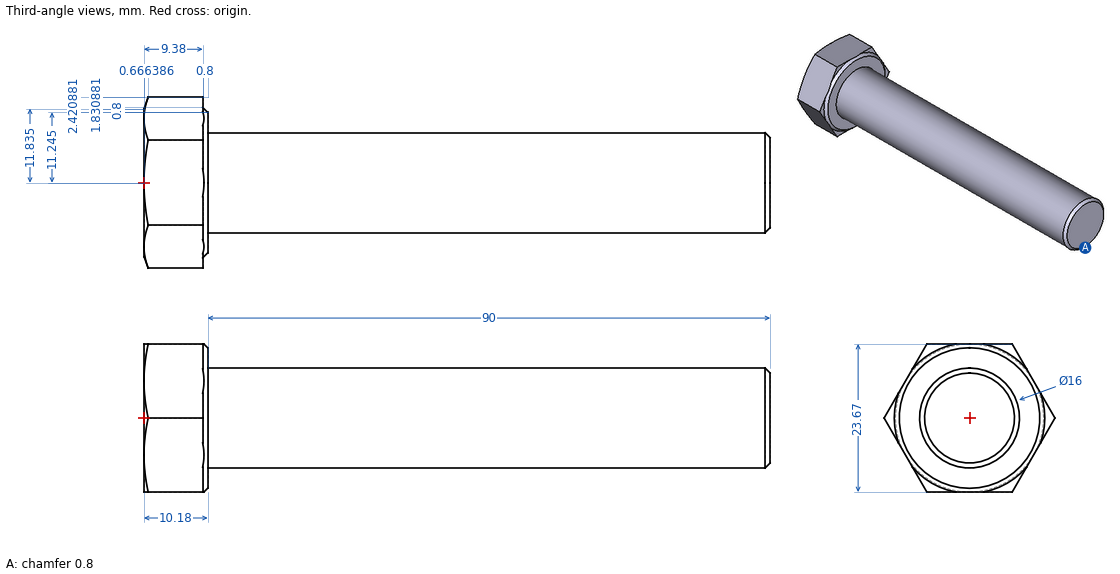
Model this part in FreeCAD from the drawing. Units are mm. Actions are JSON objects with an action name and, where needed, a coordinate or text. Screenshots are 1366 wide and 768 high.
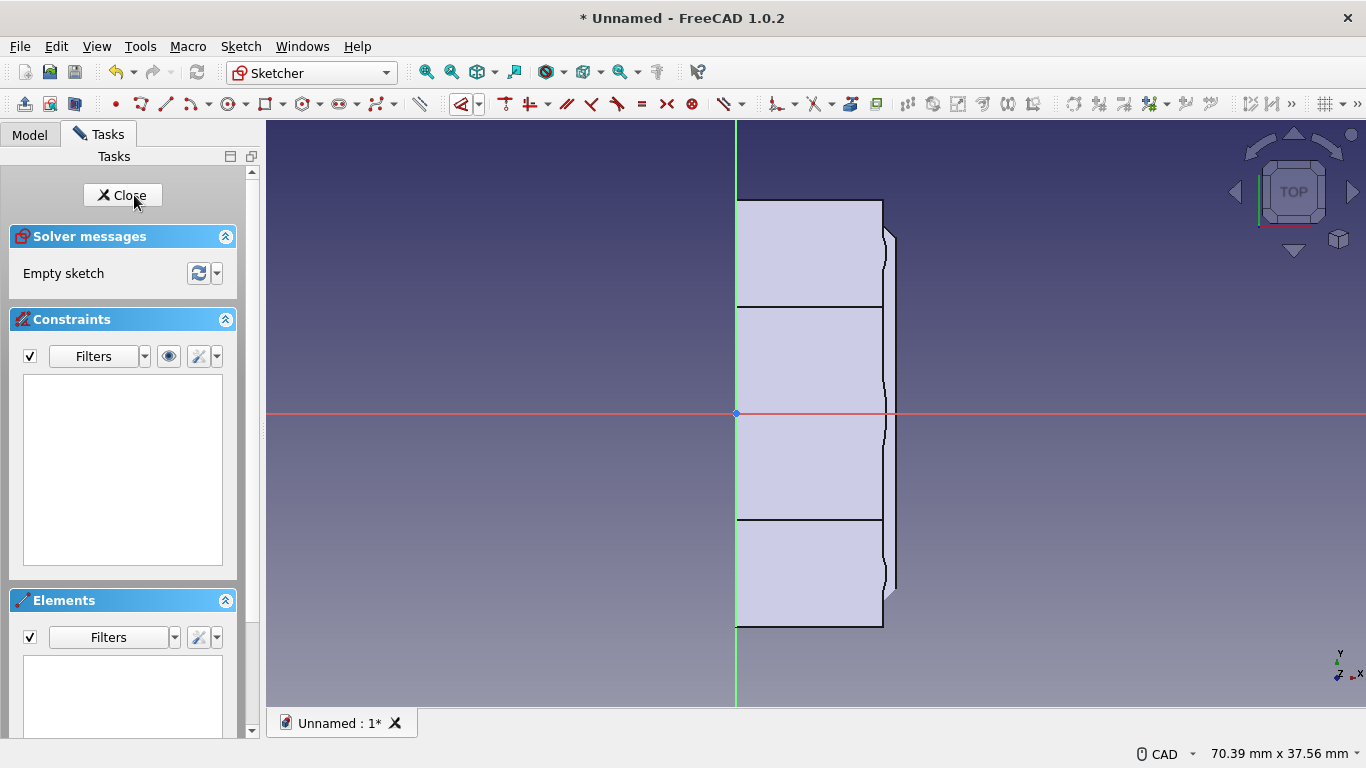
{"action": "scroll", "coordinate": [741, 198], "scroll_direction": "up", "scroll_amount": 13}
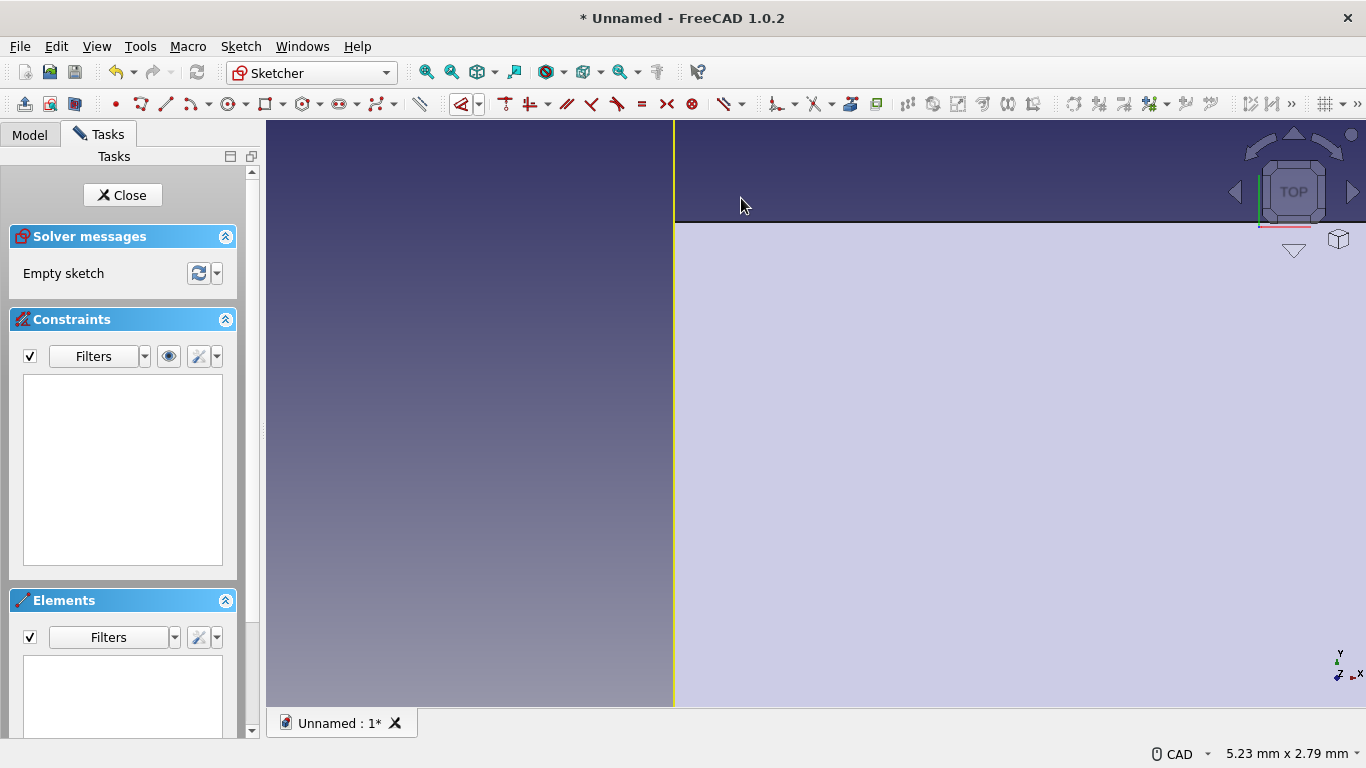
{"action": "key", "text": "g m"}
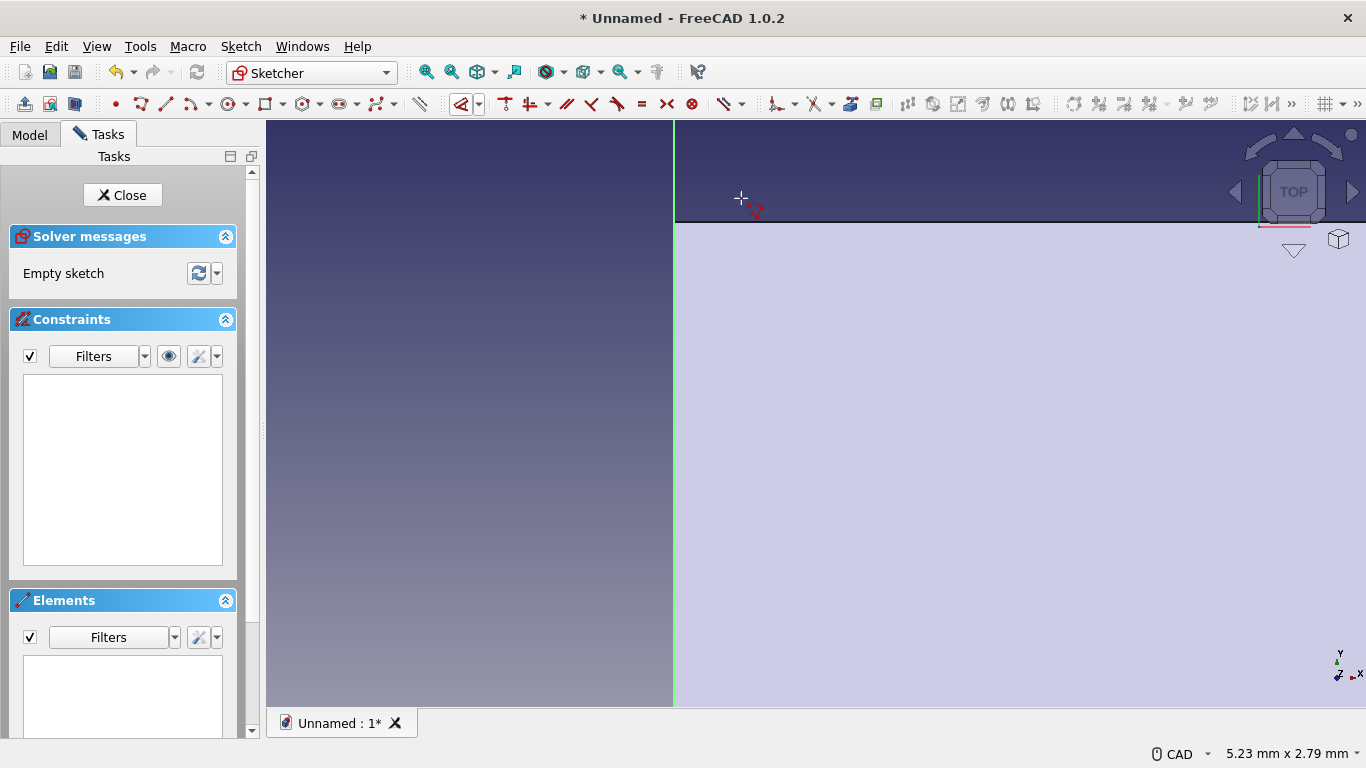
{"action": "left_click", "coordinate": [674, 608]}
{"action": "left_click", "coordinate": [815, 222]}
{"action": "left_click", "coordinate": [683, 222]}
{"action": "left_click", "coordinate": [674, 609]}
{"action": "key", "text": "Escape"}
{"action": "key", "text": "Escape"}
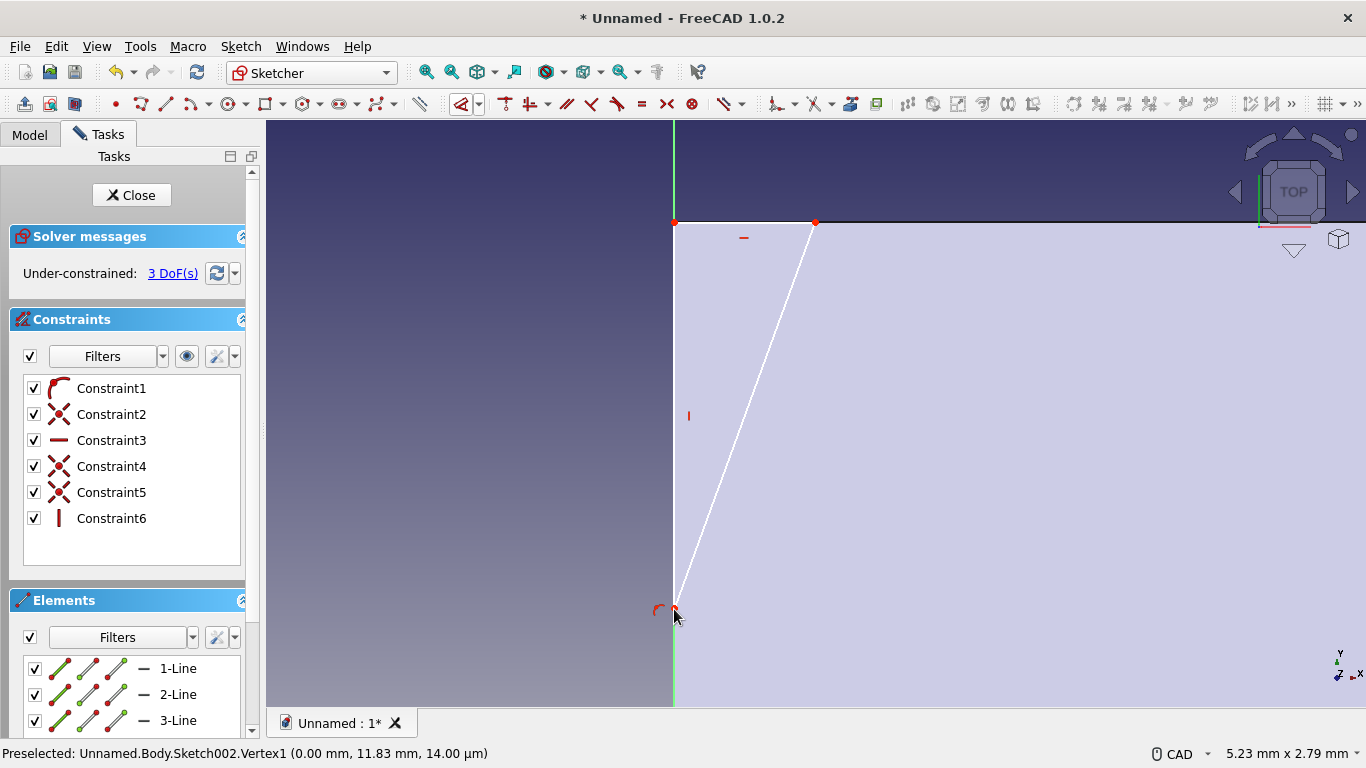
{"action": "left_click", "coordinate": [674, 609]}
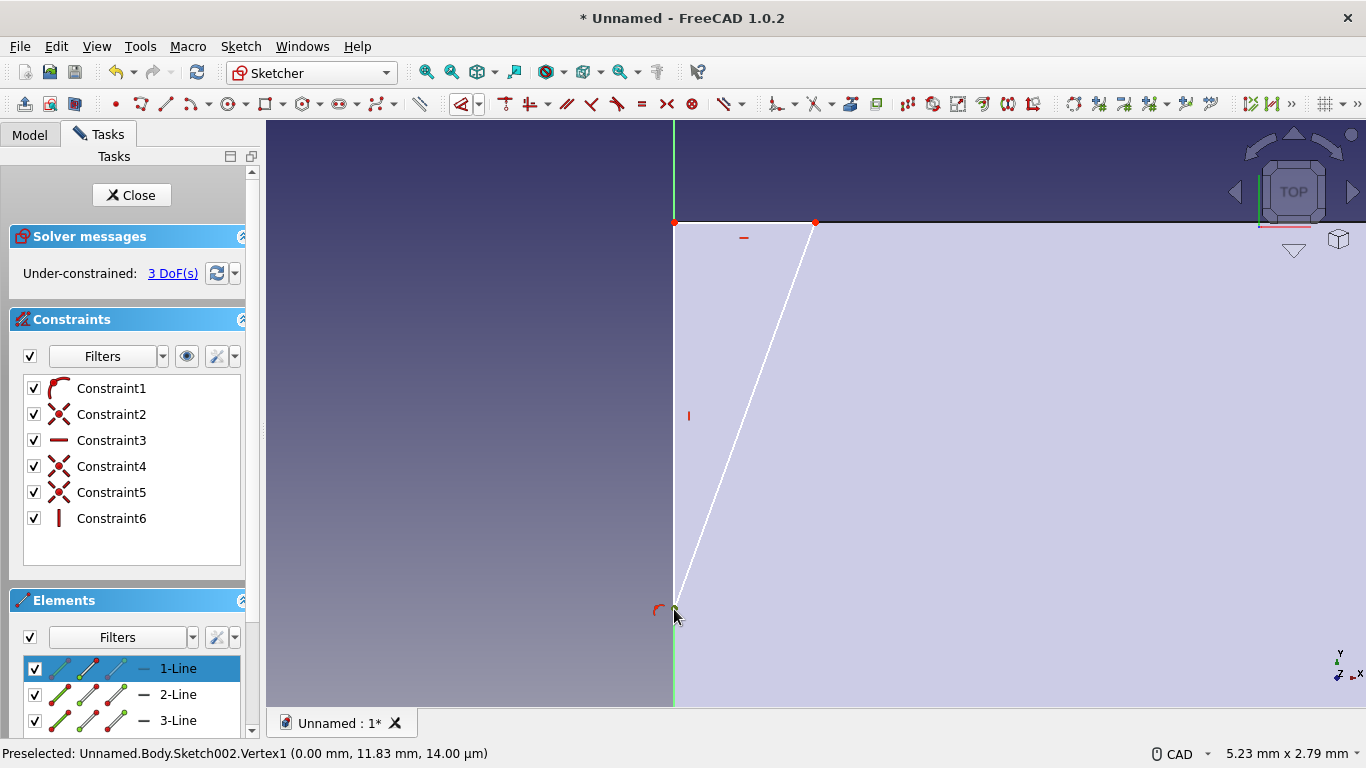
{"action": "key", "text": "i"}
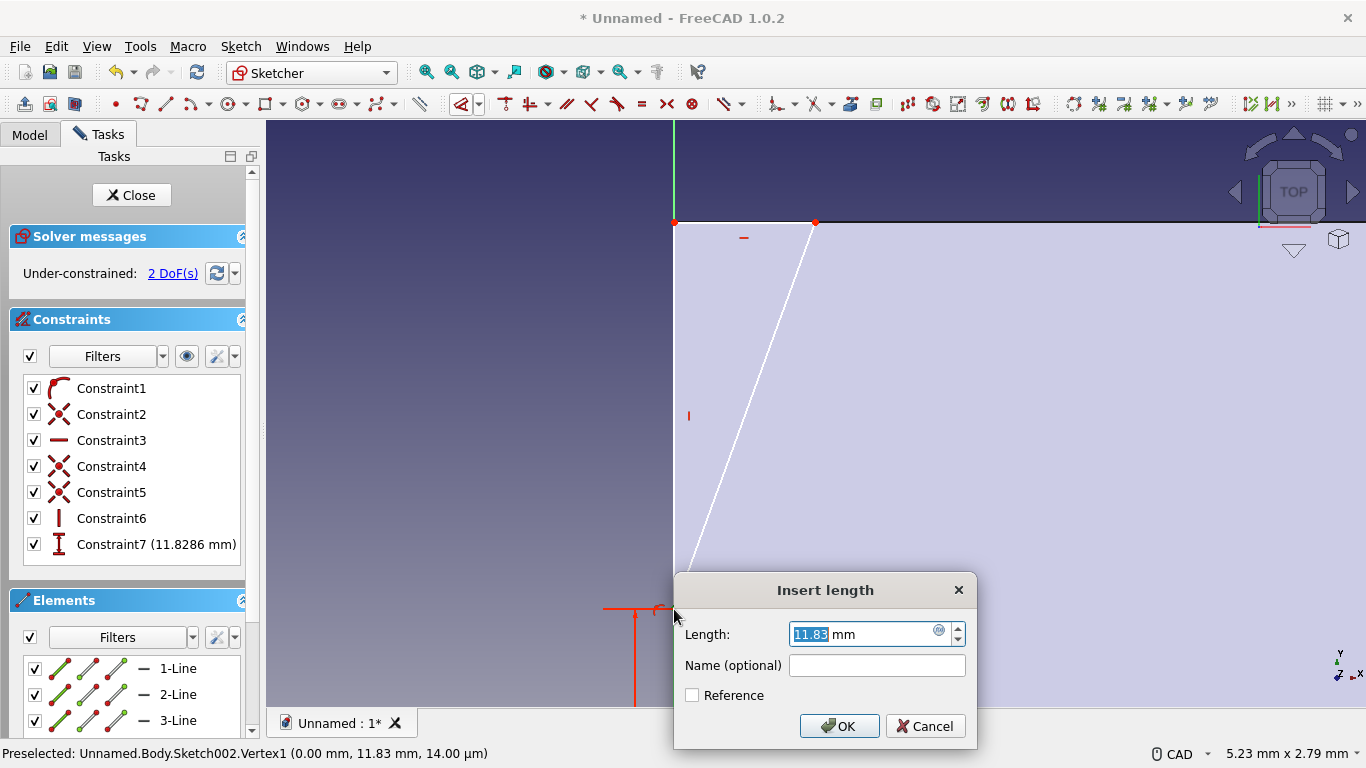
{"action": "type", "text": "11.835"}
{"action": "key", "text": "Return"}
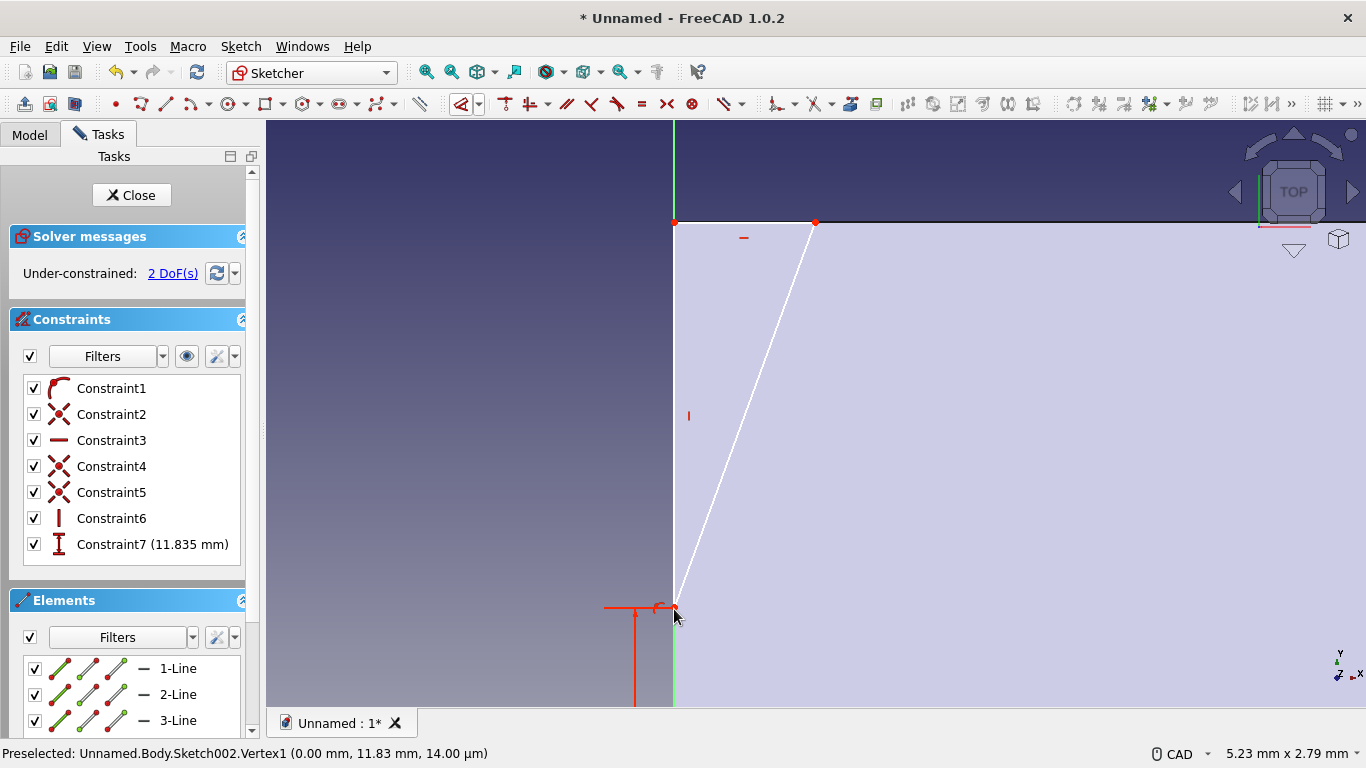
{"action": "left_click", "coordinate": [773, 223]}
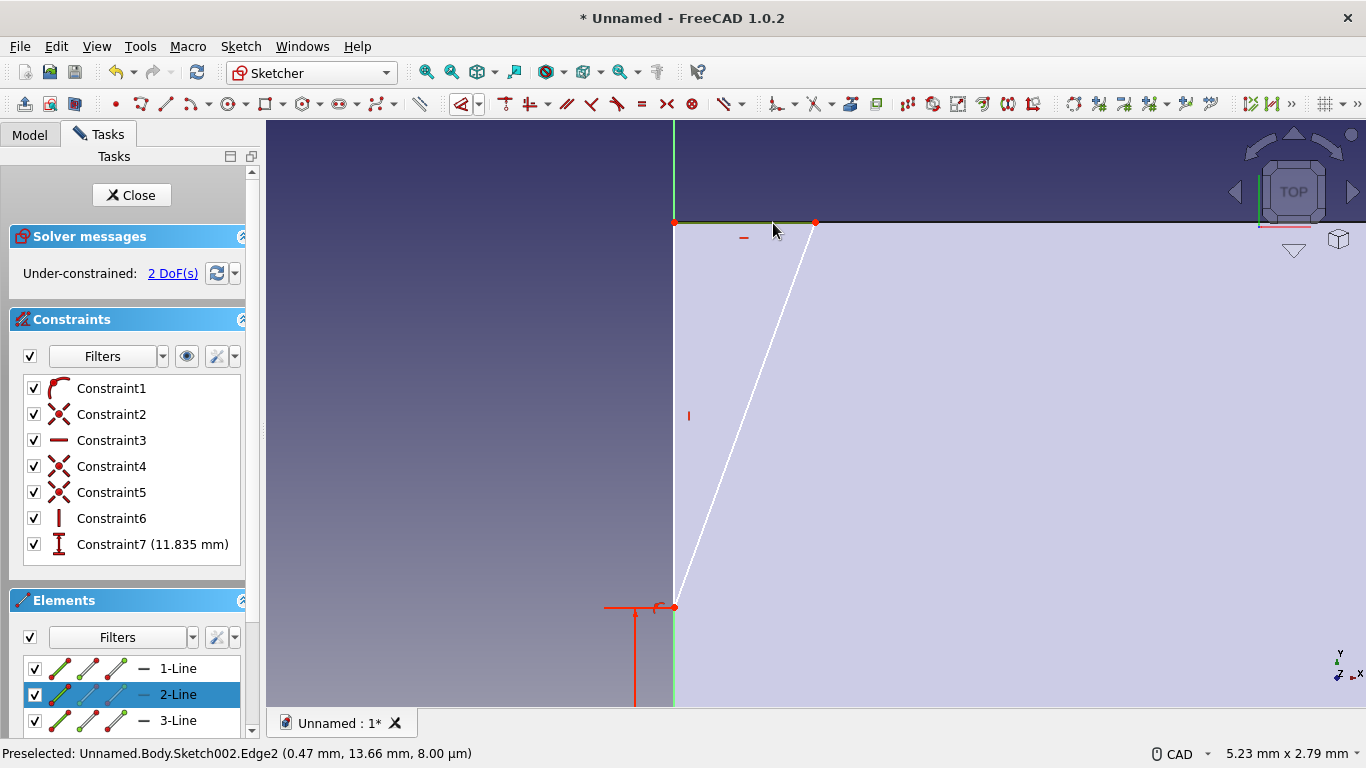
{"action": "key", "text": "l"}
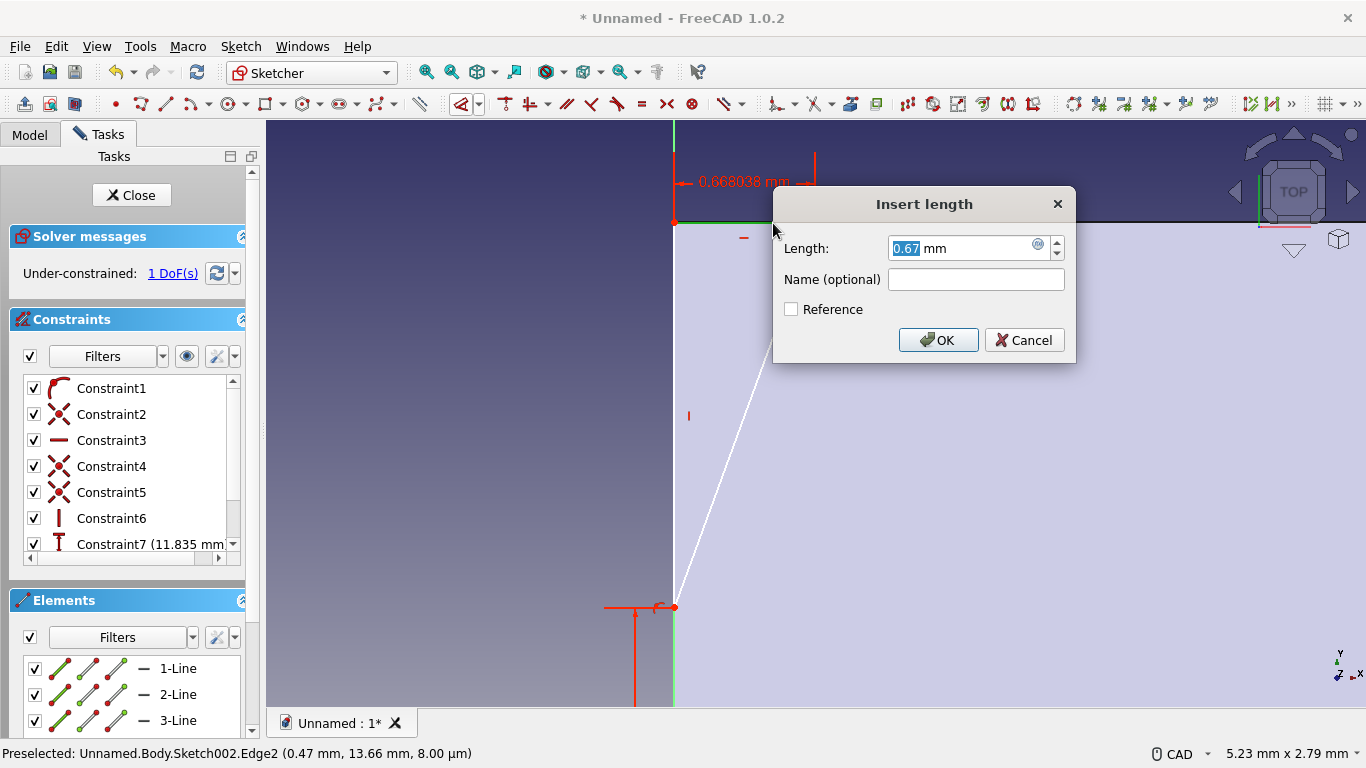
{"action": "type", "text": "0.666386"}
{"action": "key", "text": "Return"}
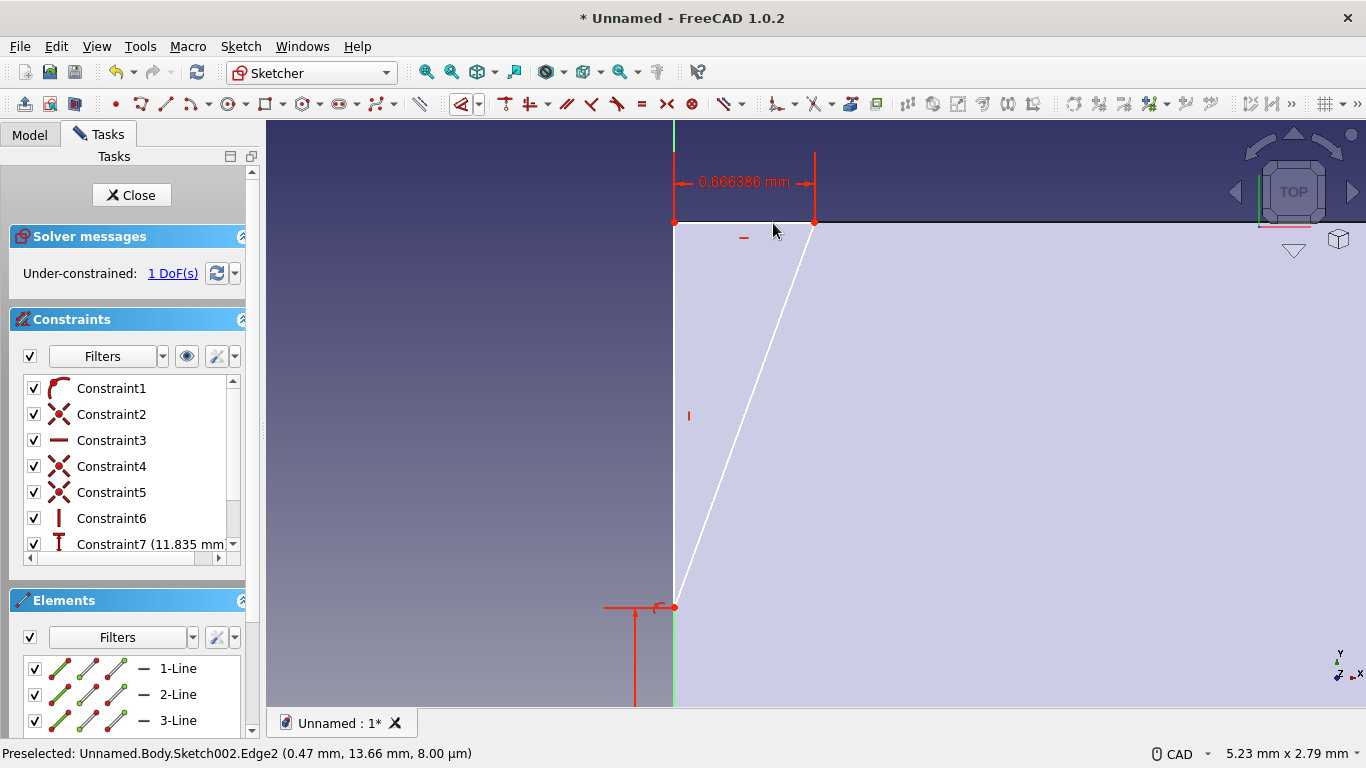
{"action": "left_click", "coordinate": [674, 338]}